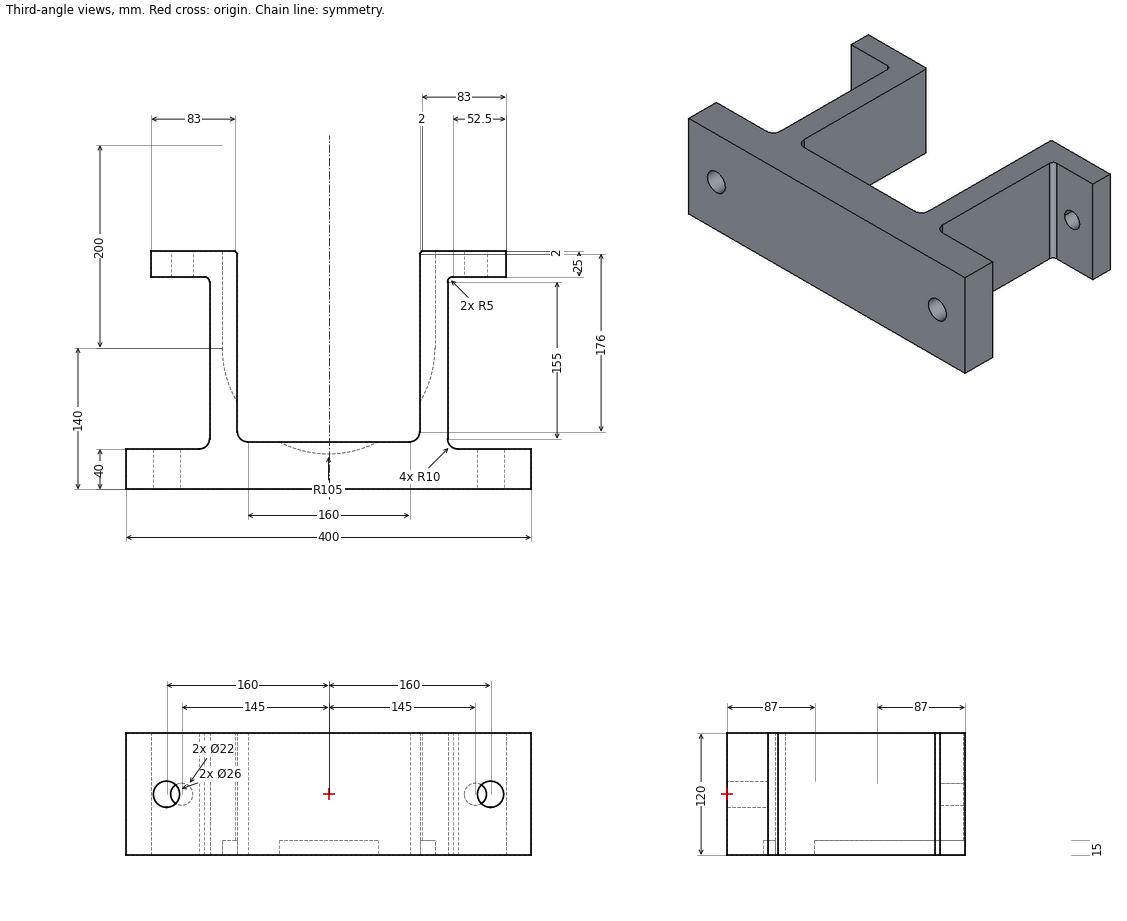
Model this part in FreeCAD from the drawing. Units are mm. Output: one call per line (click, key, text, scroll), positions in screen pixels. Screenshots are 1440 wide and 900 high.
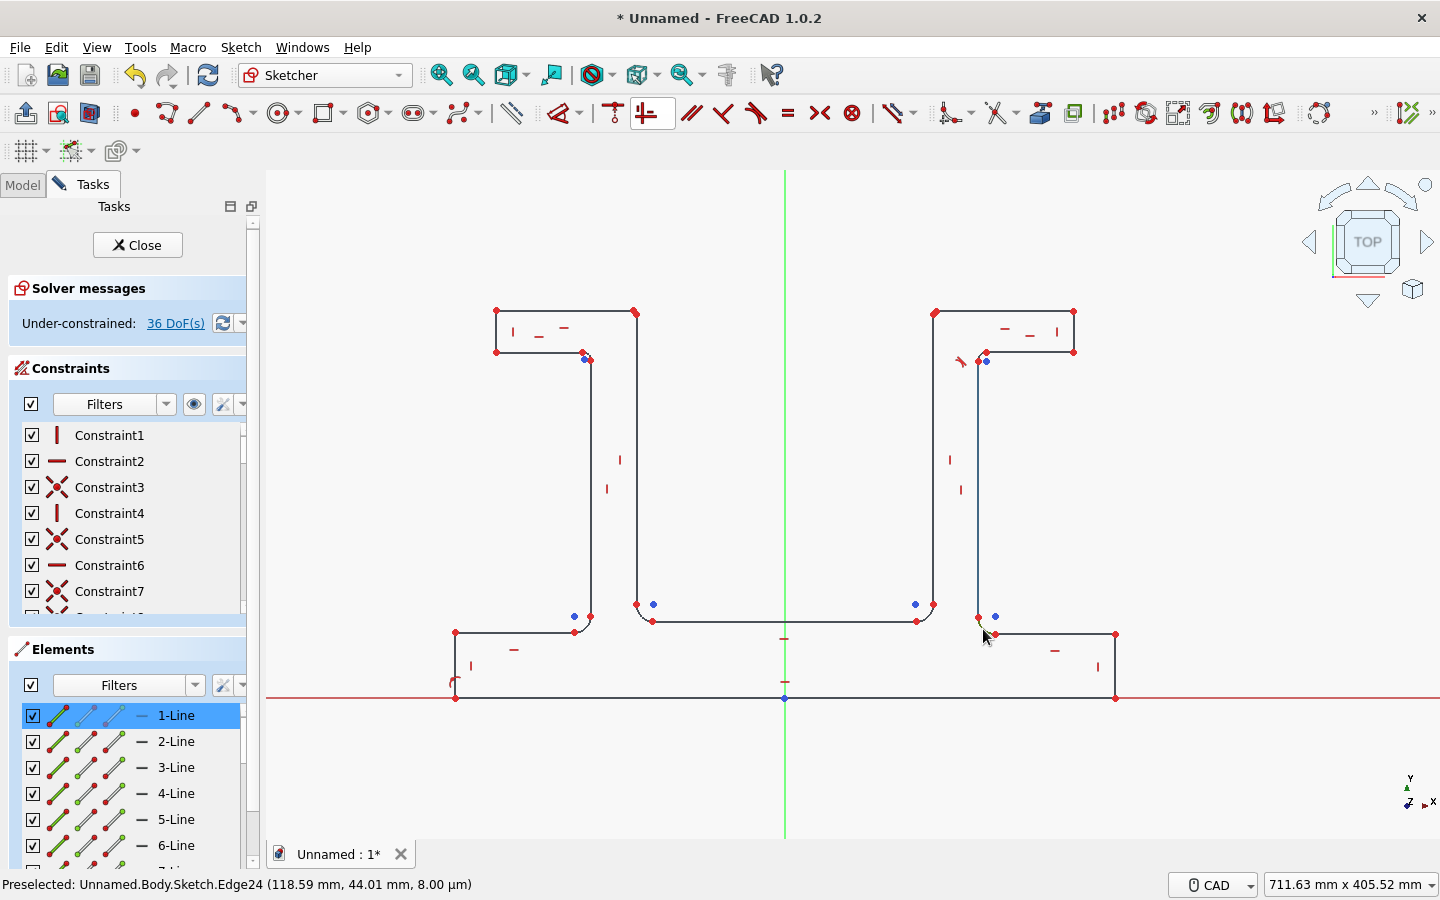
click(756, 114)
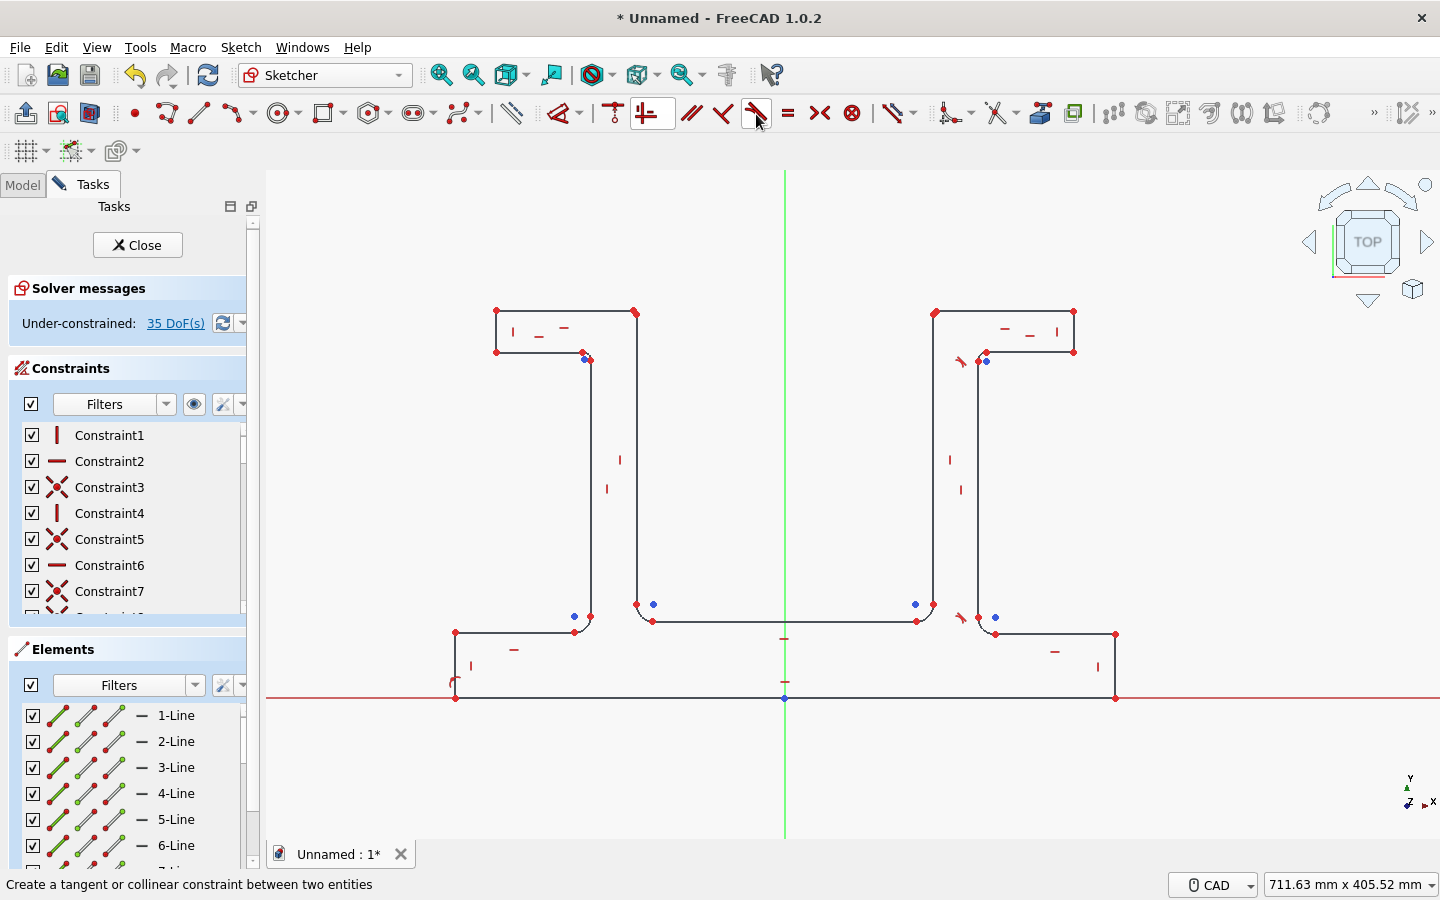
click(1013, 352)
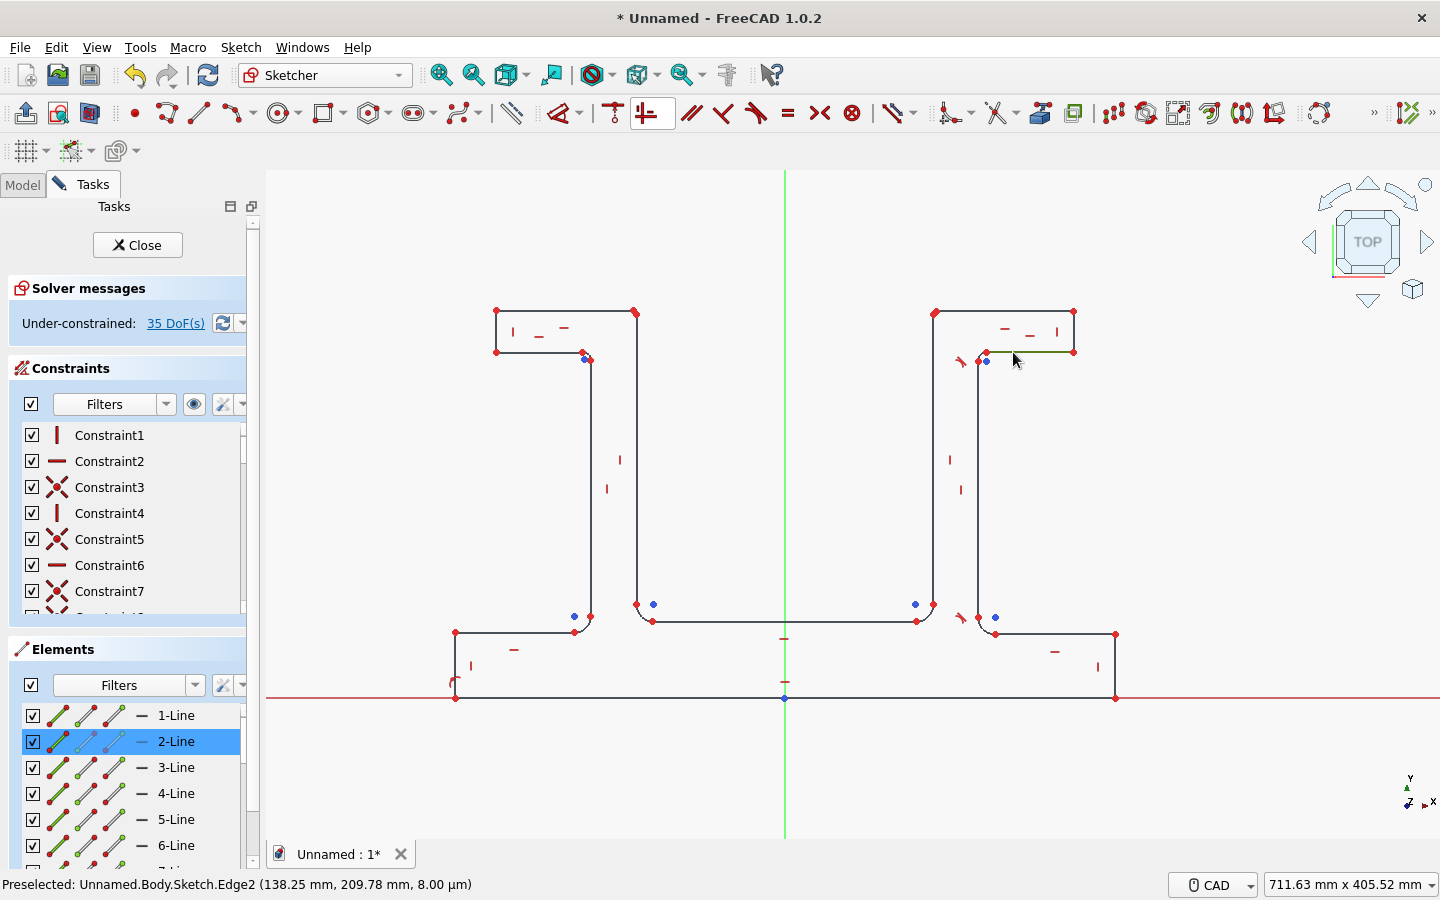
scroll(981, 355, up, 4)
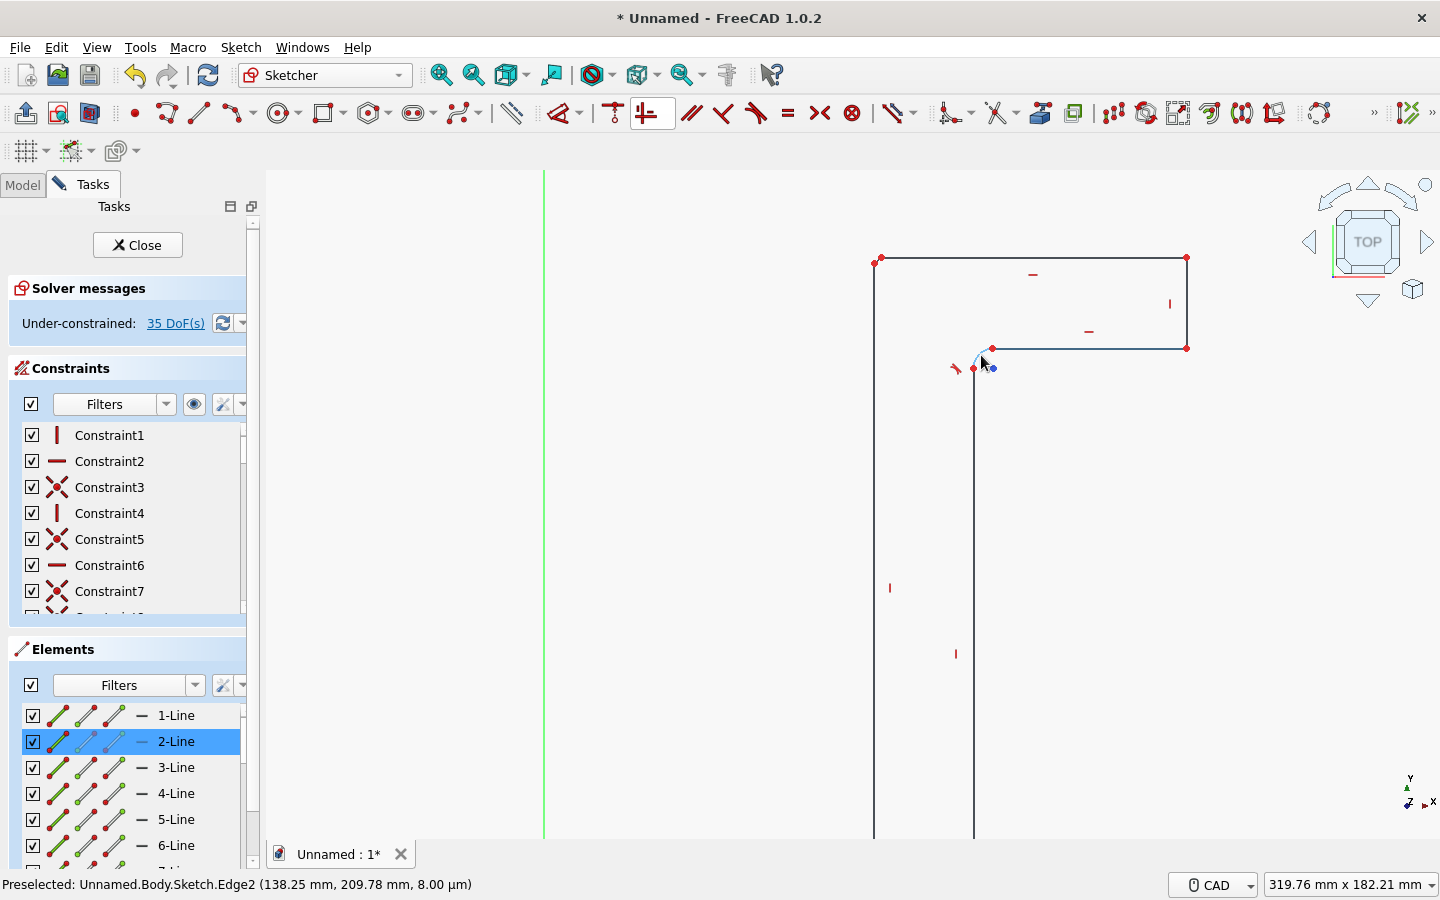
click(979, 354)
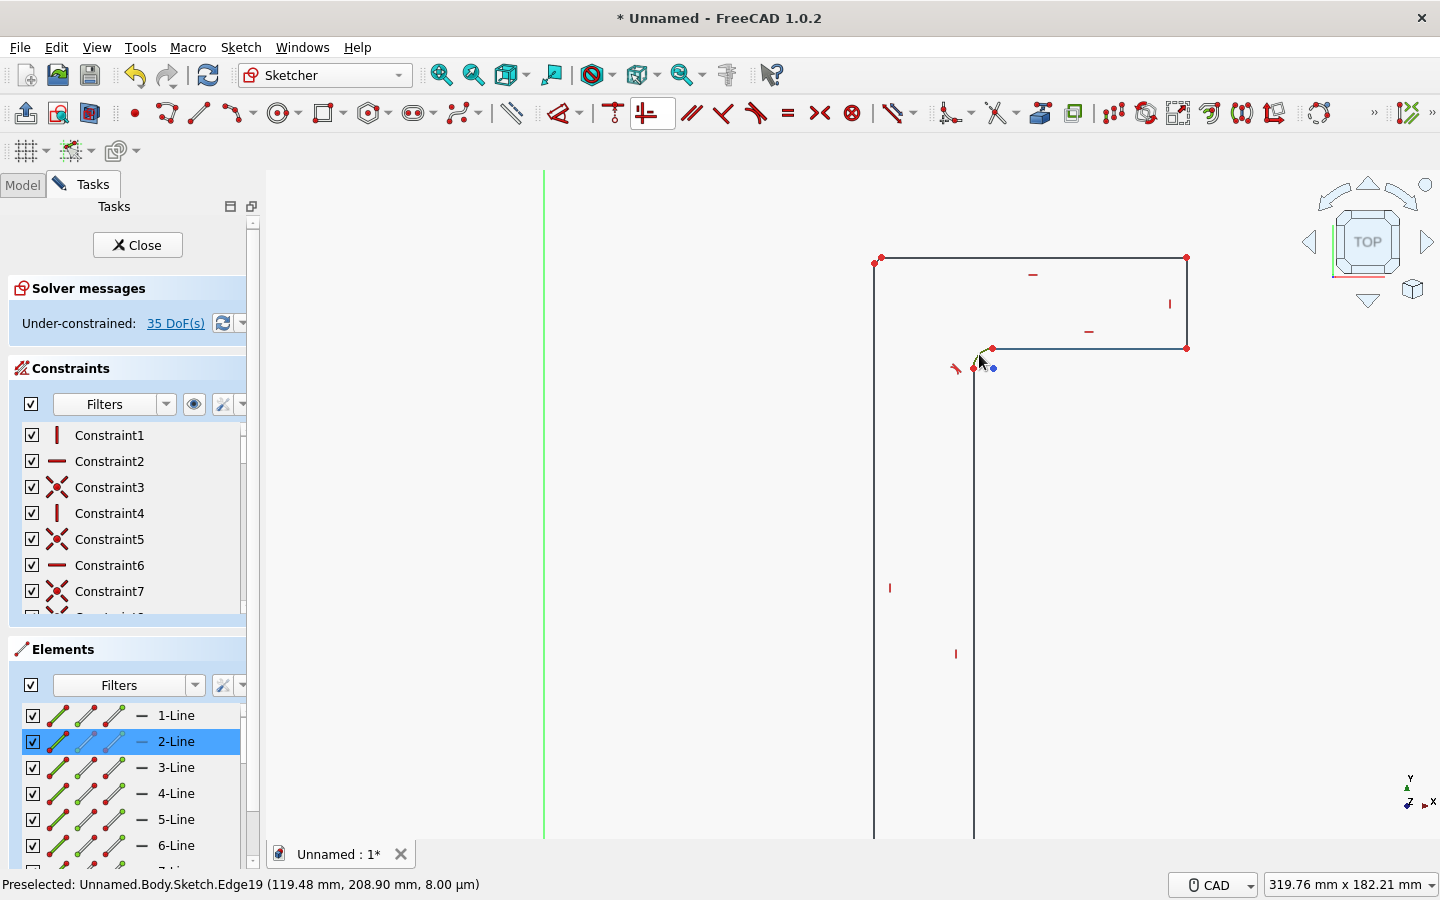
click(756, 114)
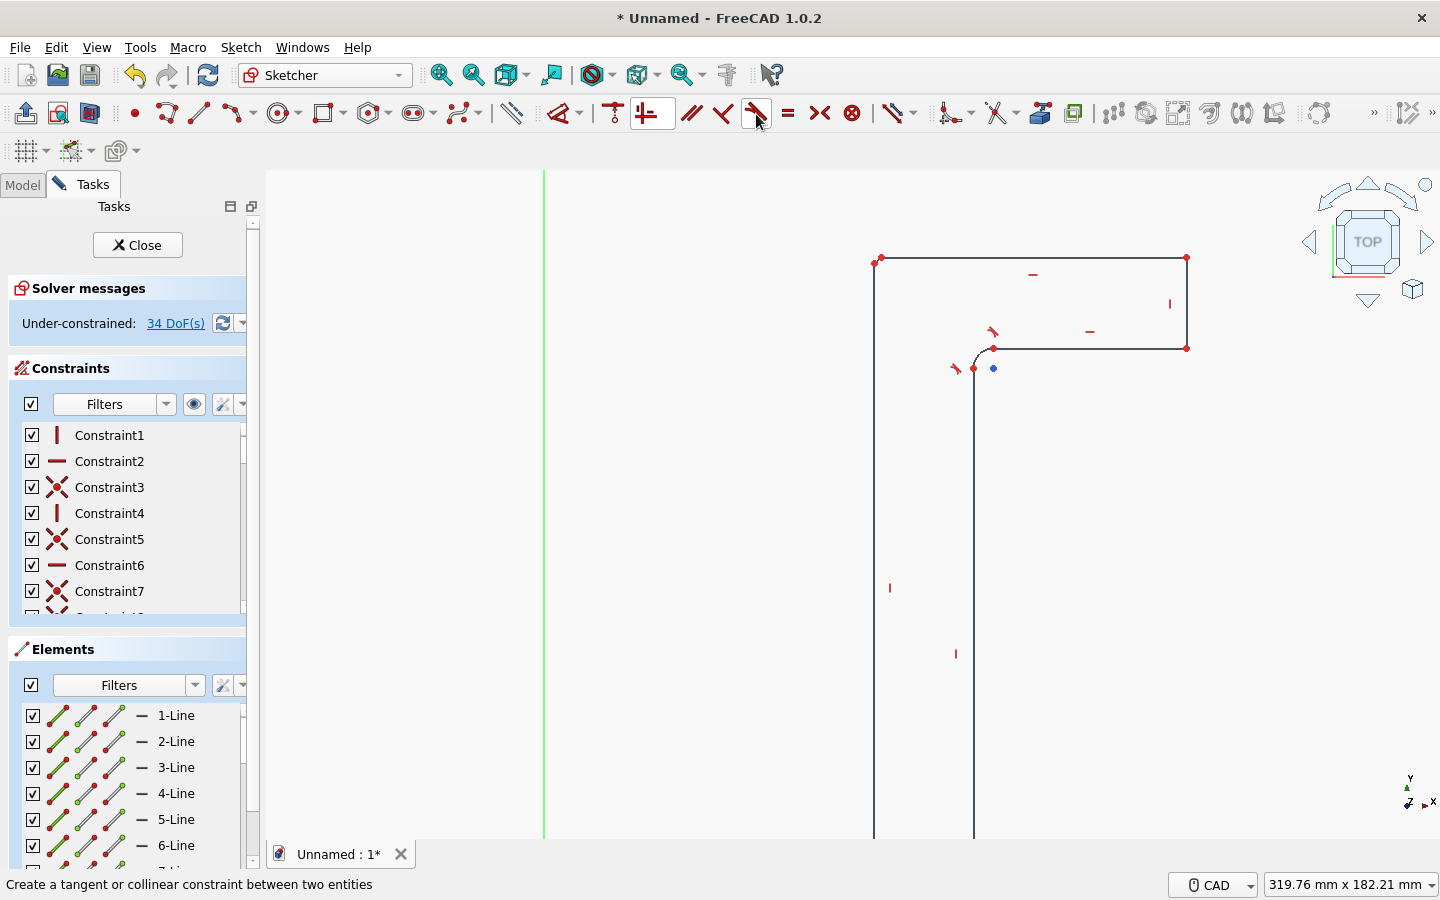
click(874, 458)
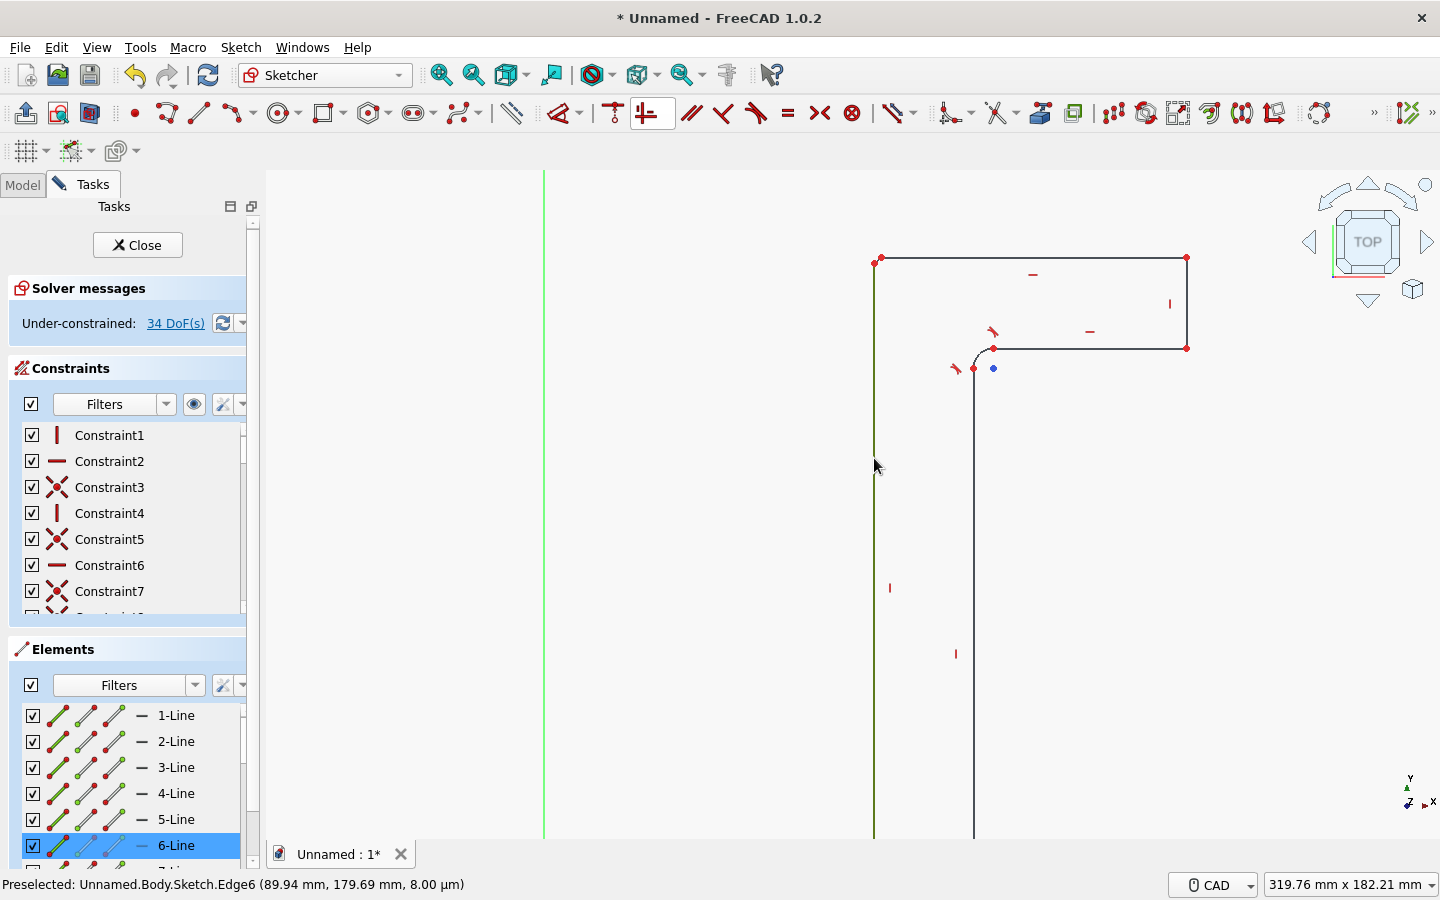
scroll(981, 355, down, 4)